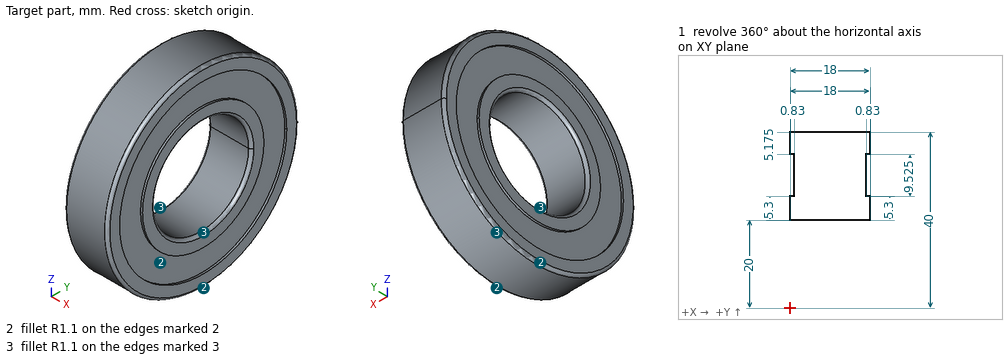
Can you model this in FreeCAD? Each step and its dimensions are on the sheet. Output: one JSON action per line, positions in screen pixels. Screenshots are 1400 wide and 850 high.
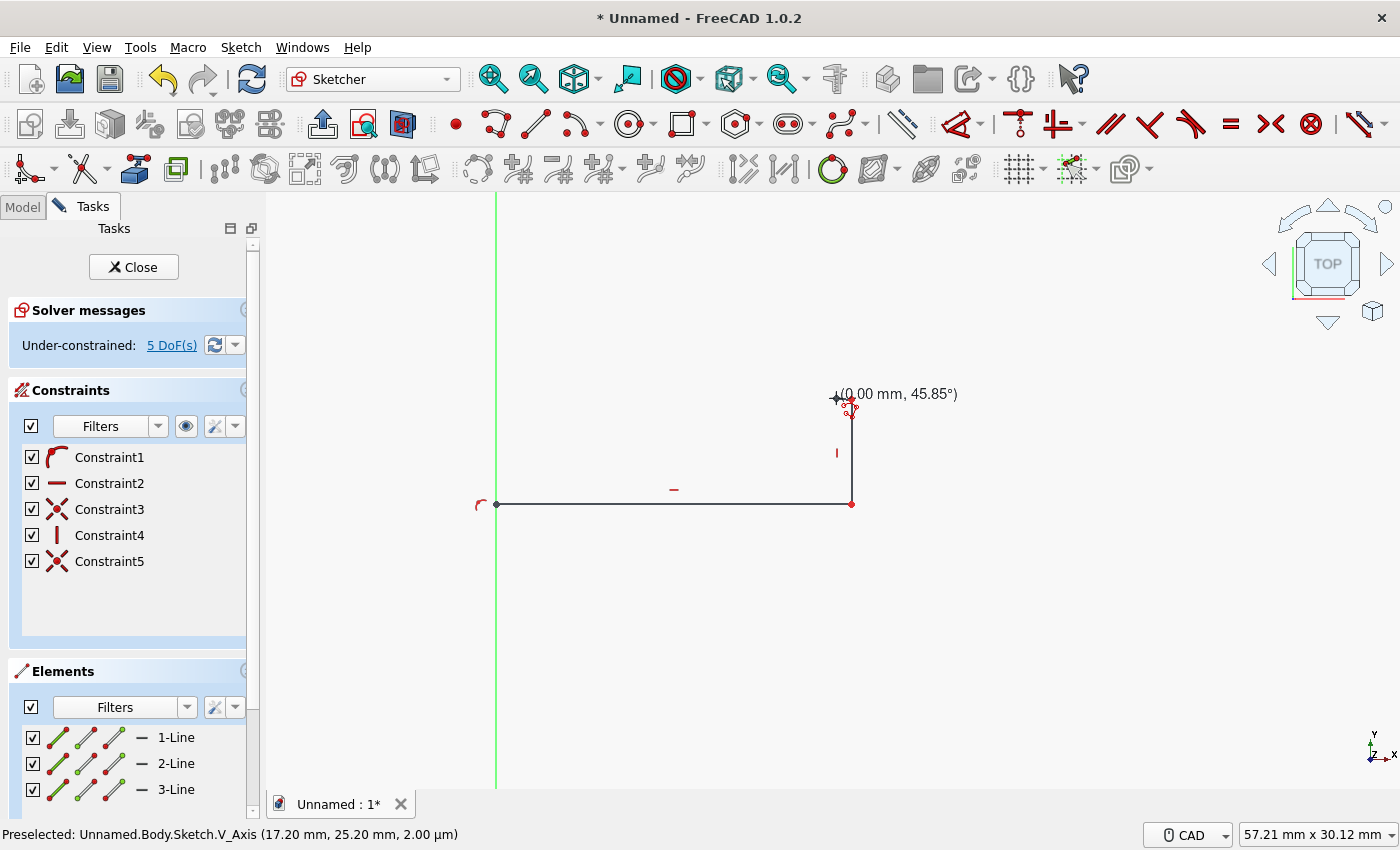
{"action": "scroll", "coordinate": [838, 480], "scroll_direction": "down", "scroll_amount": 4}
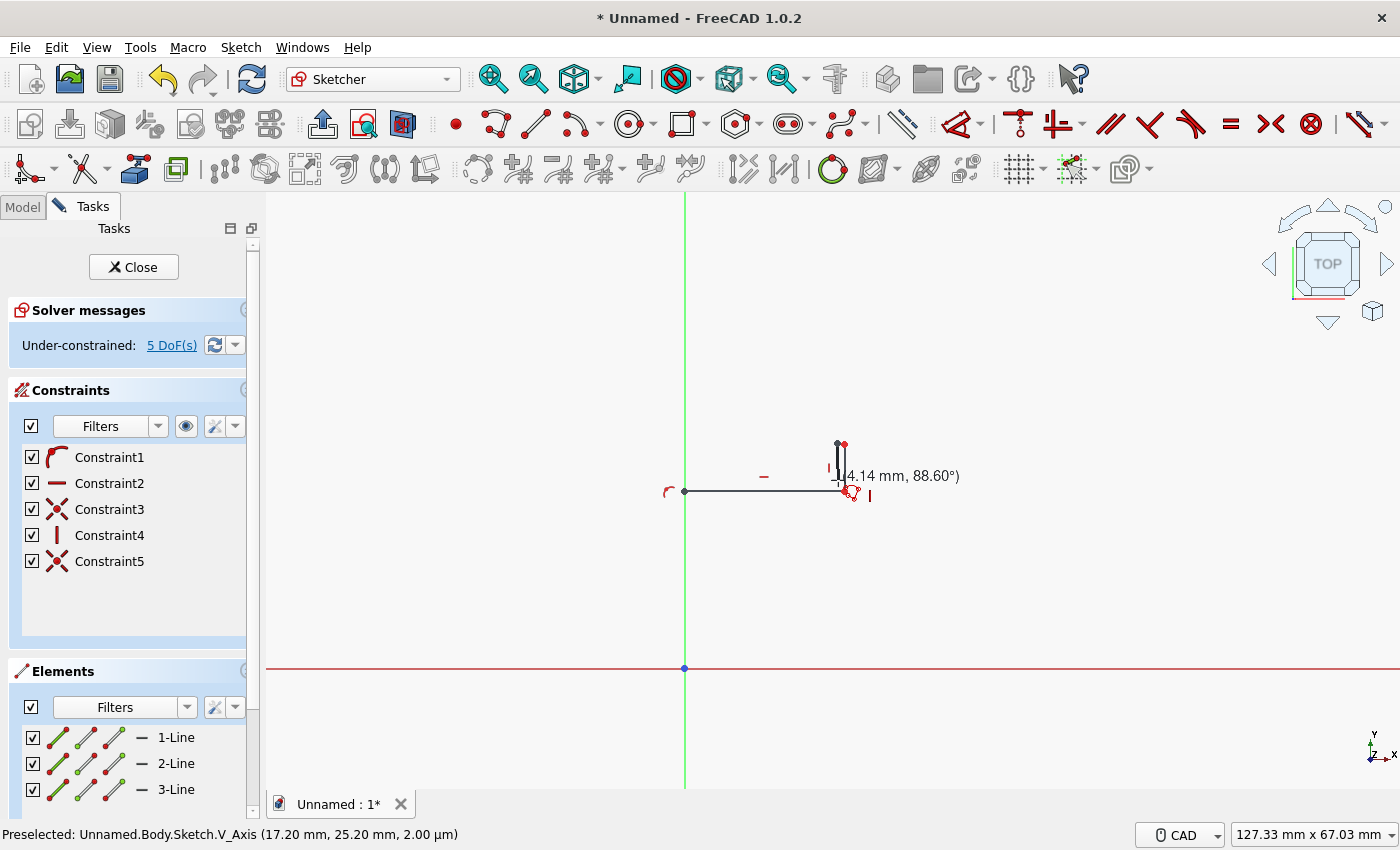
{"action": "left_click", "coordinate": [837, 359]}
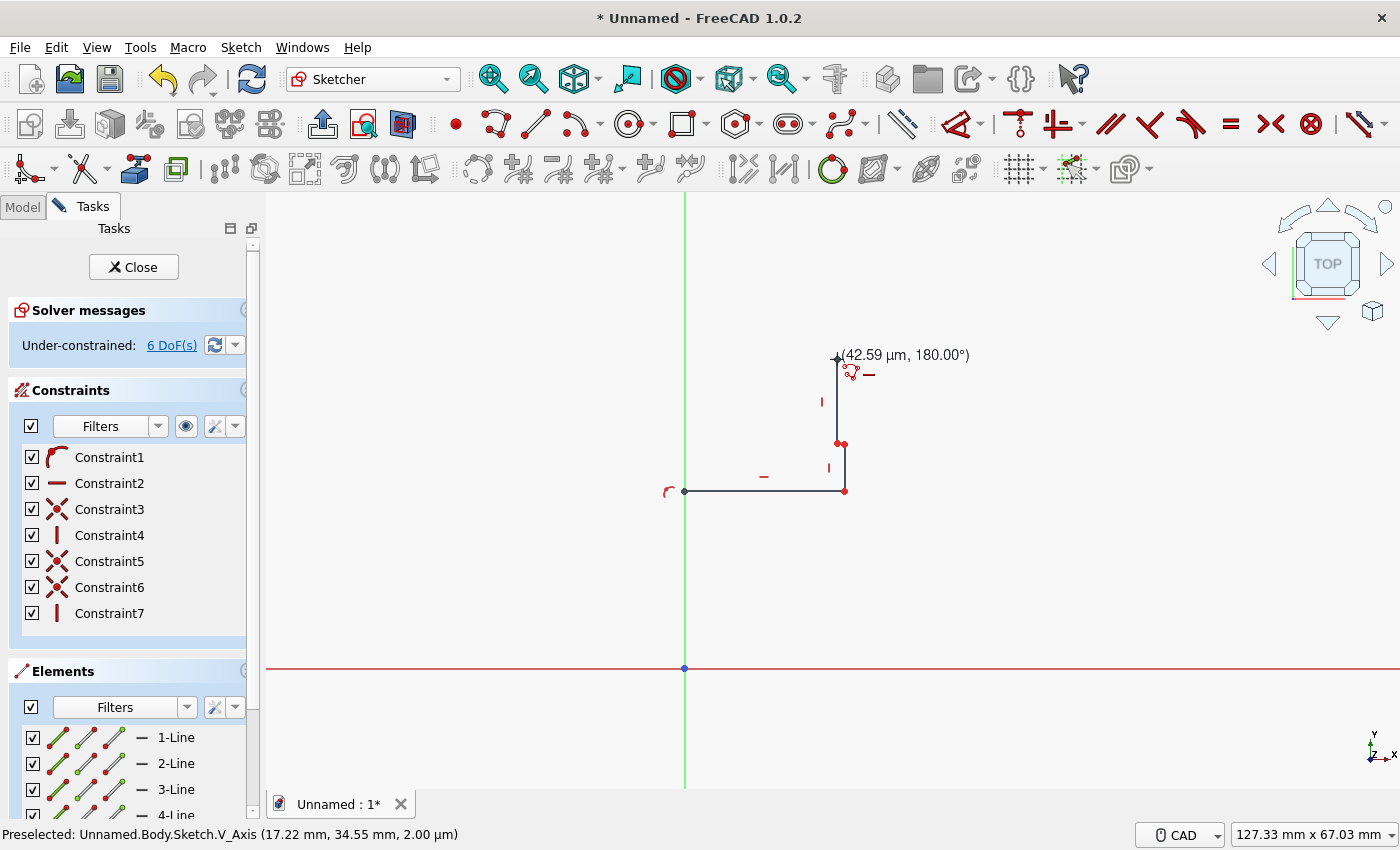
{"action": "scroll", "coordinate": [845, 359], "scroll_direction": "up", "scroll_amount": 4}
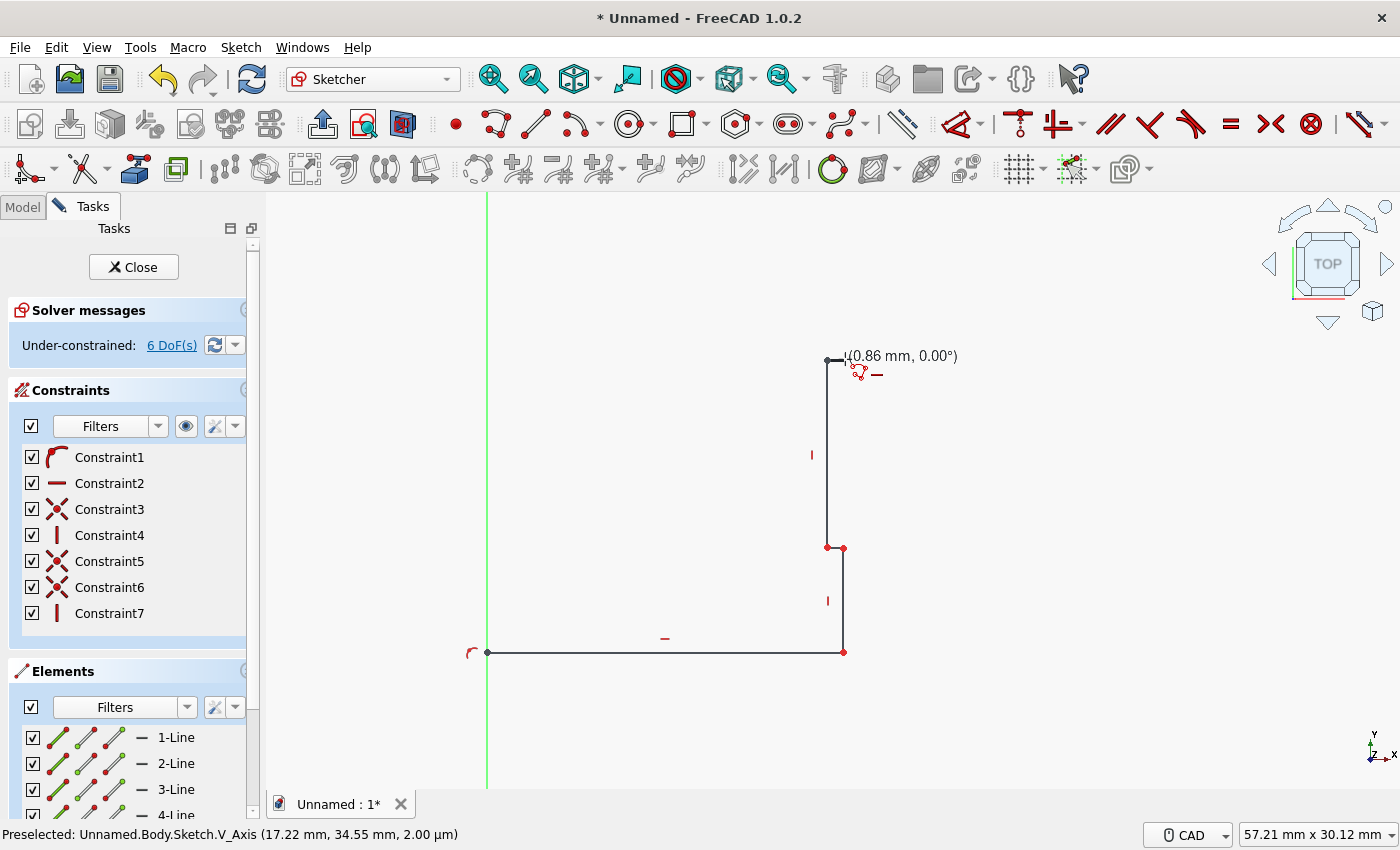
{"action": "left_click", "coordinate": [844, 359]}
{"action": "left_click", "coordinate": [844, 255]}
{"action": "left_click", "coordinate": [487, 255]}
{"action": "left_click", "coordinate": [496, 358]}
{"action": "left_click", "coordinate": [504, 358]}
{"action": "left_click", "coordinate": [504, 547]}
{"action": "left_click", "coordinate": [496, 547]}
{"action": "left_click", "coordinate": [487, 653]}
{"action": "key", "text": "Escape"}
{"action": "key", "text": "Escape"}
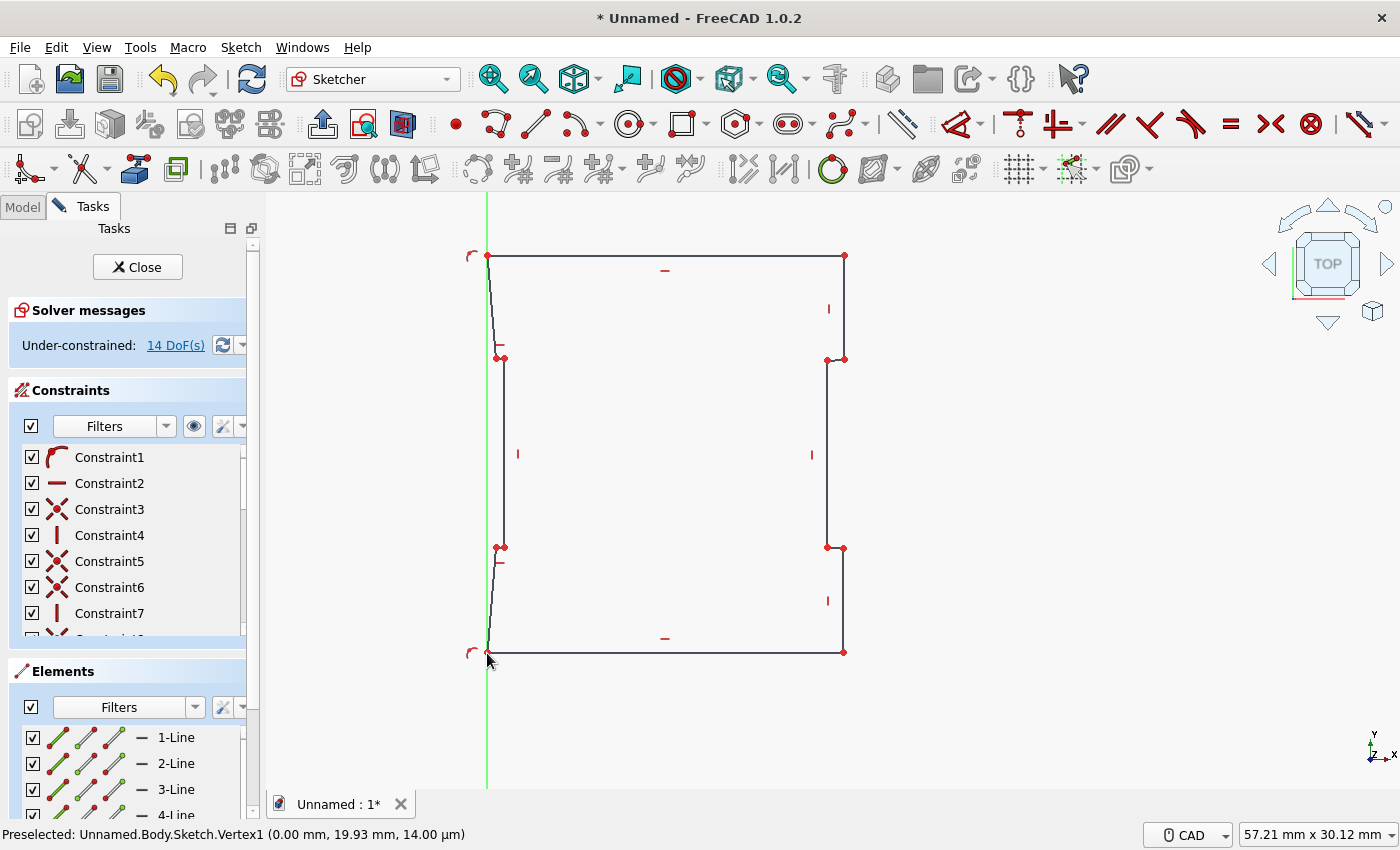
{"action": "scroll", "coordinate": [835, 548], "scroll_direction": "up", "scroll_amount": 3}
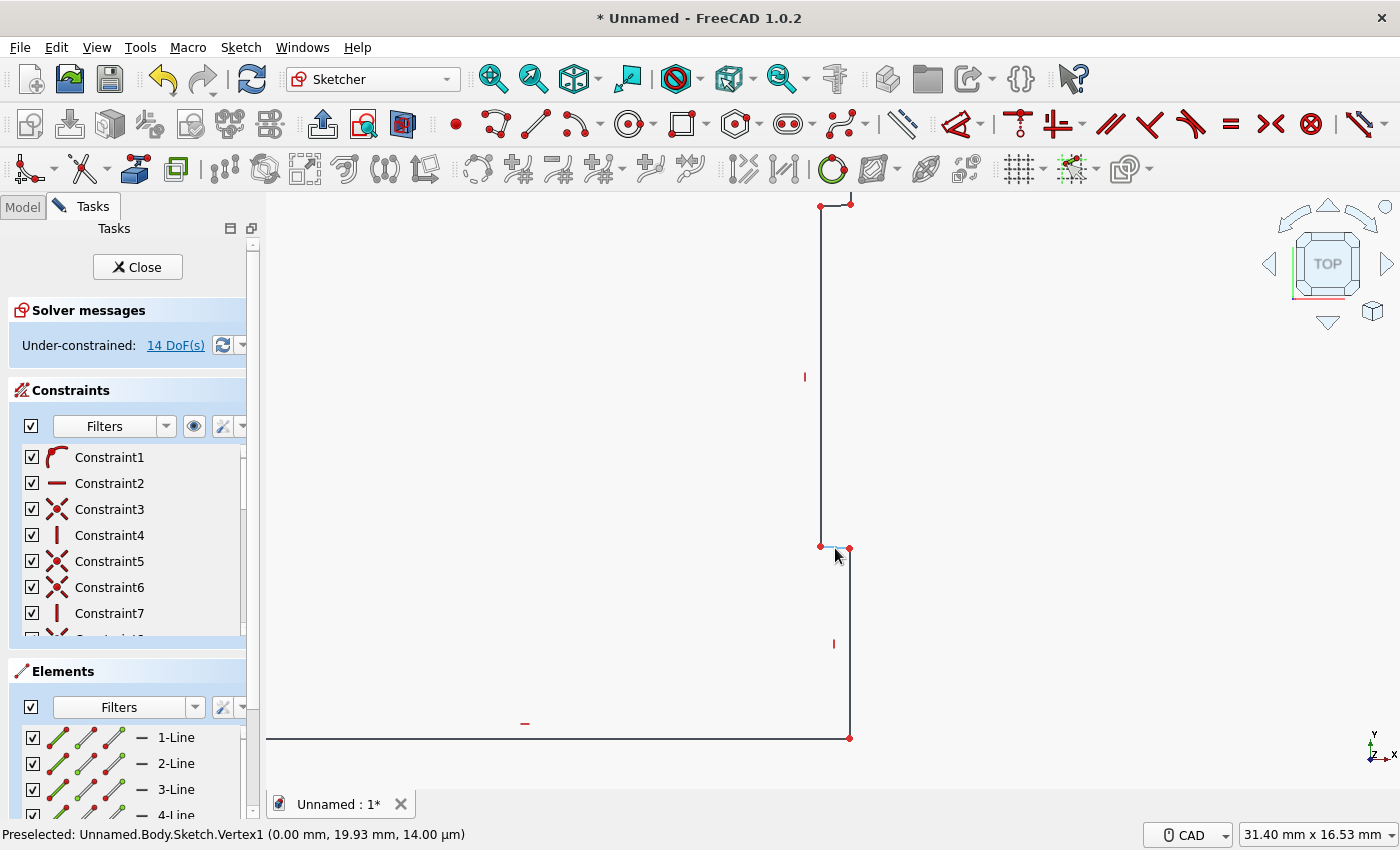
{"action": "left_click", "coordinate": [835, 547]}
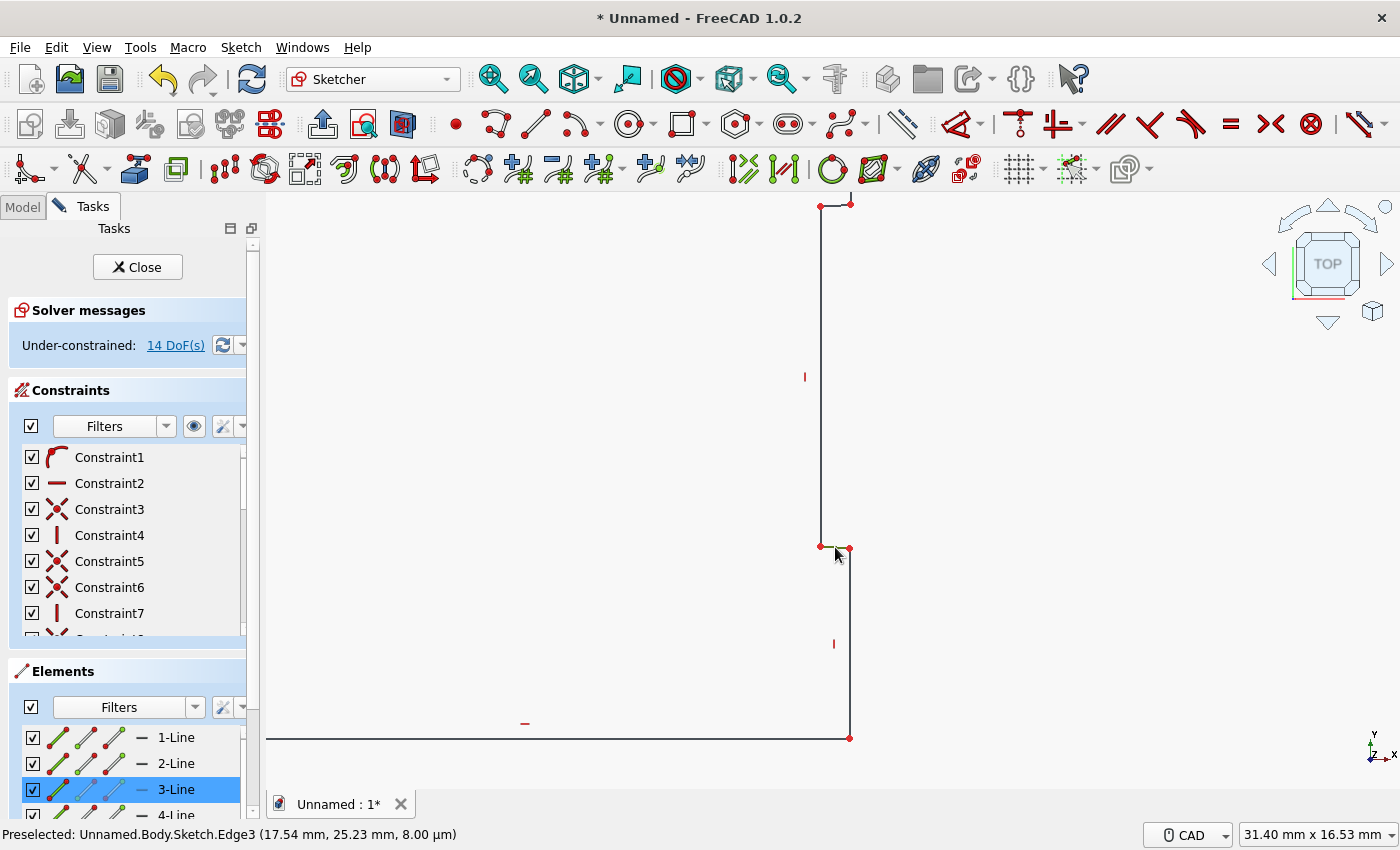
{"action": "key", "text": "h"}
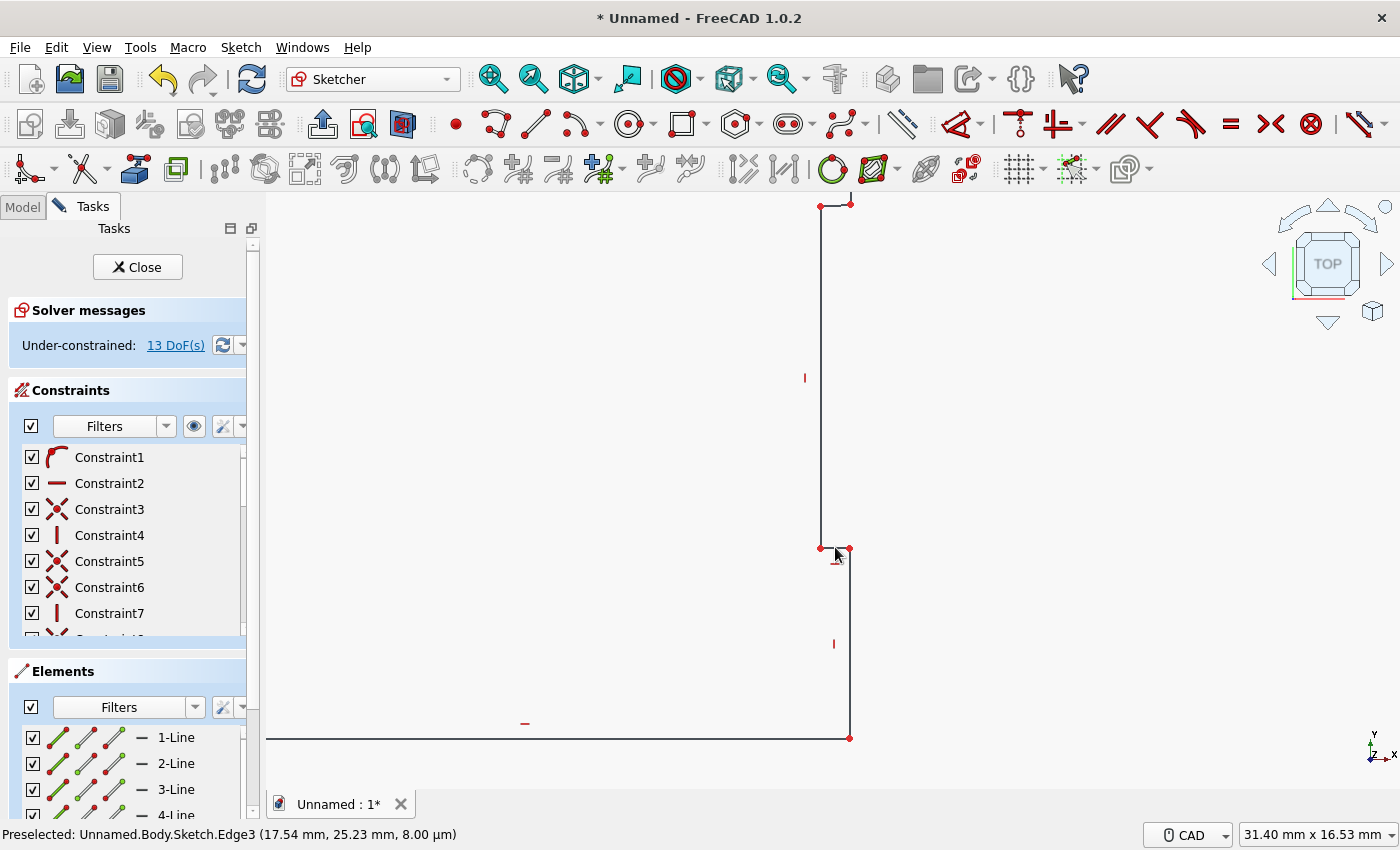
{"action": "scroll", "coordinate": [842, 410], "scroll_direction": "down", "scroll_amount": 7}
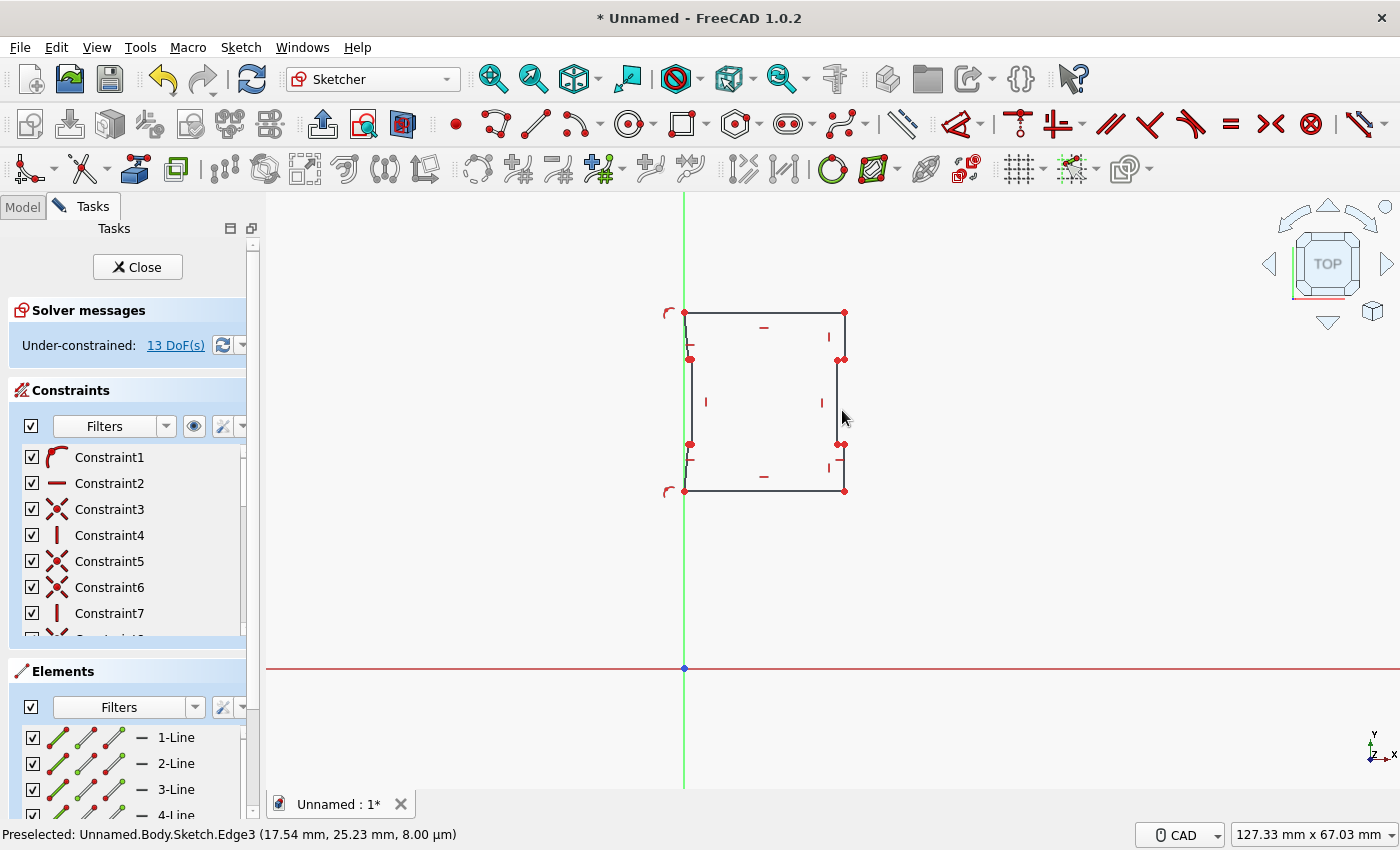
{"action": "scroll", "coordinate": [839, 360], "scroll_direction": "up", "scroll_amount": 10}